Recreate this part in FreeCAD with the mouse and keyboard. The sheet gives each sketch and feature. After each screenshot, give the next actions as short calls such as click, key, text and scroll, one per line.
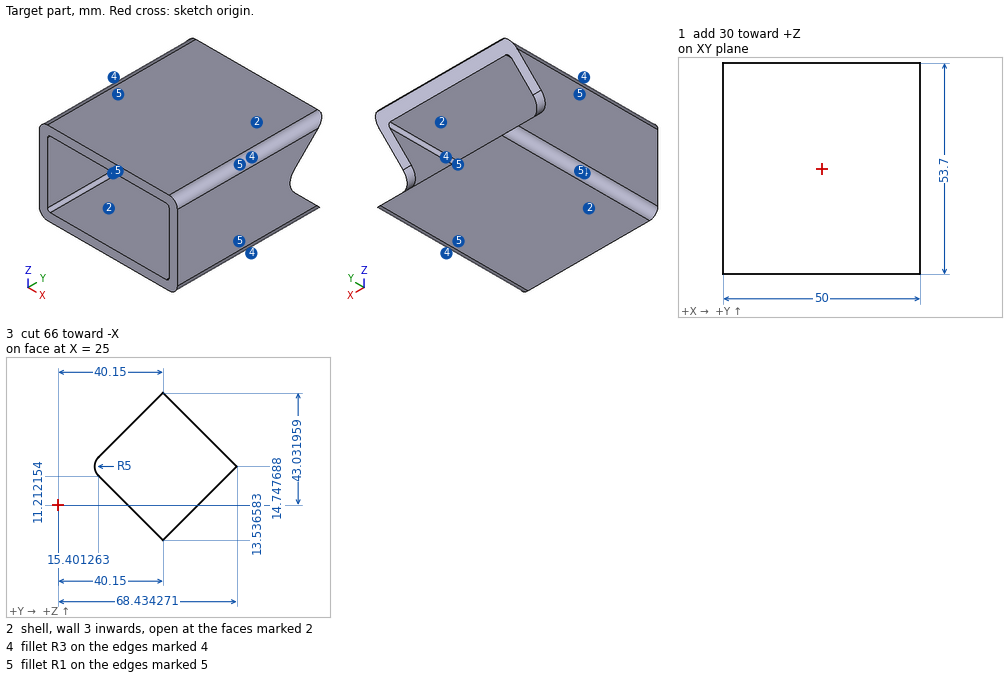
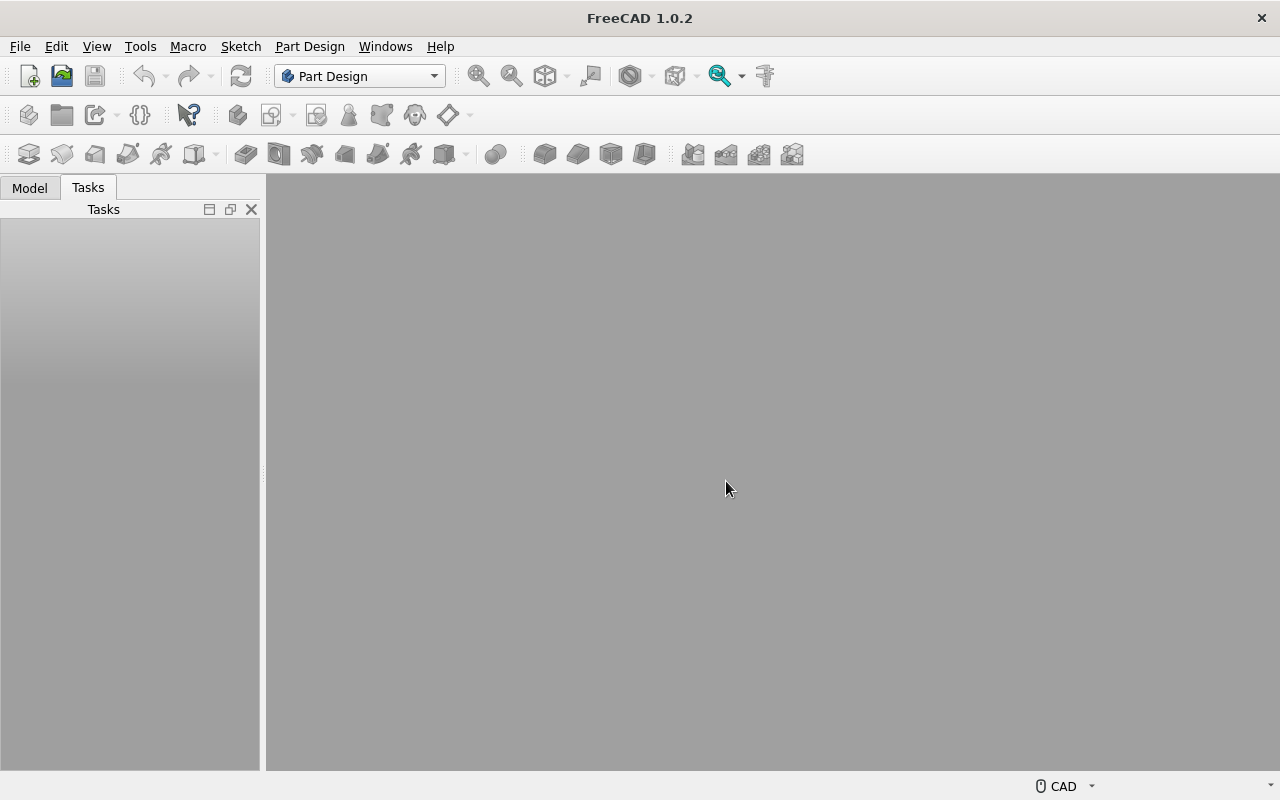
key(ctrl+n)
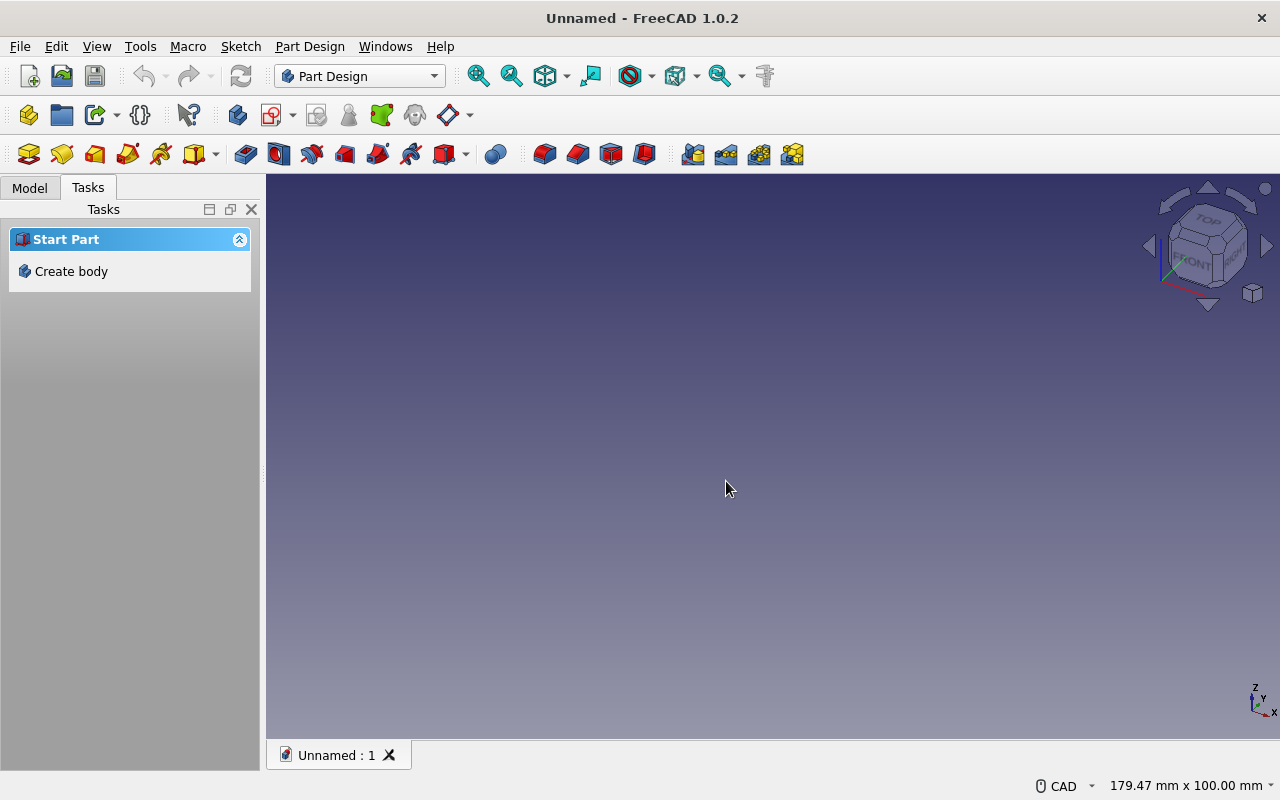
click(270, 116)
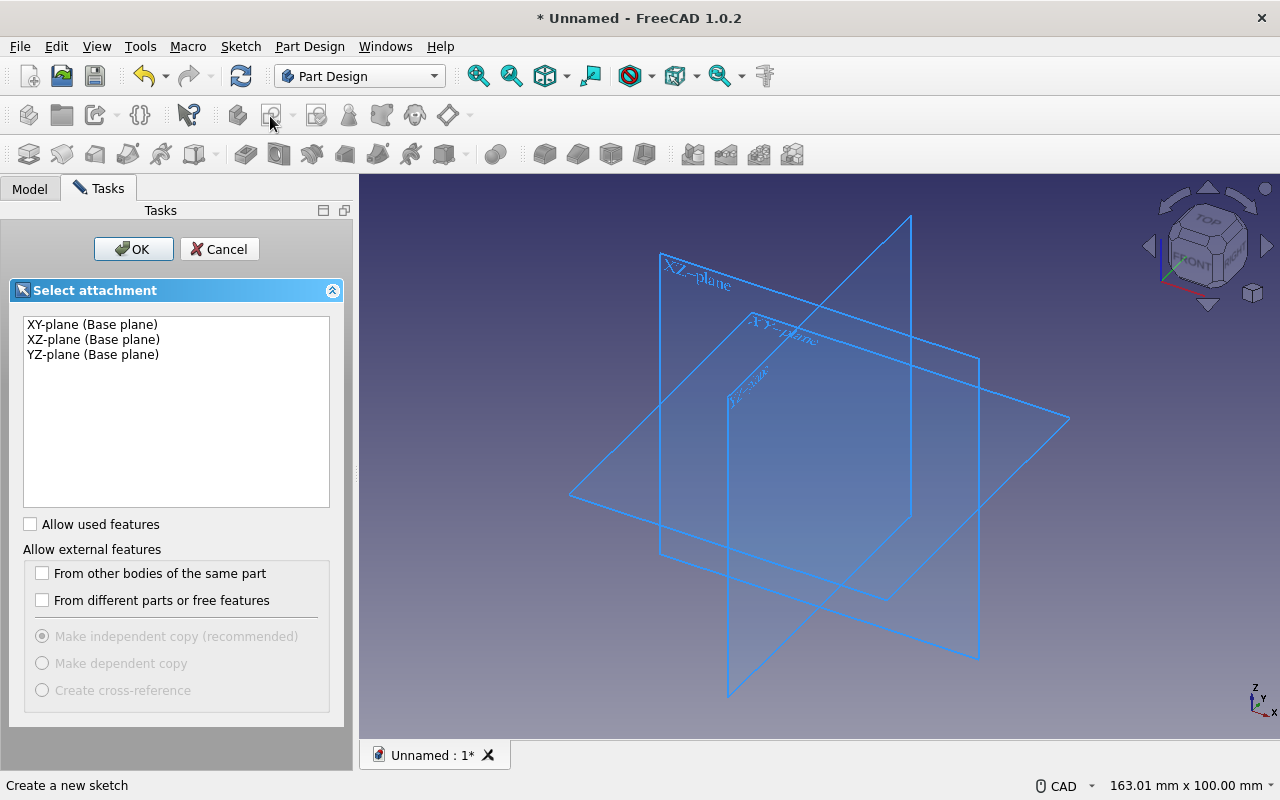
click(84, 324)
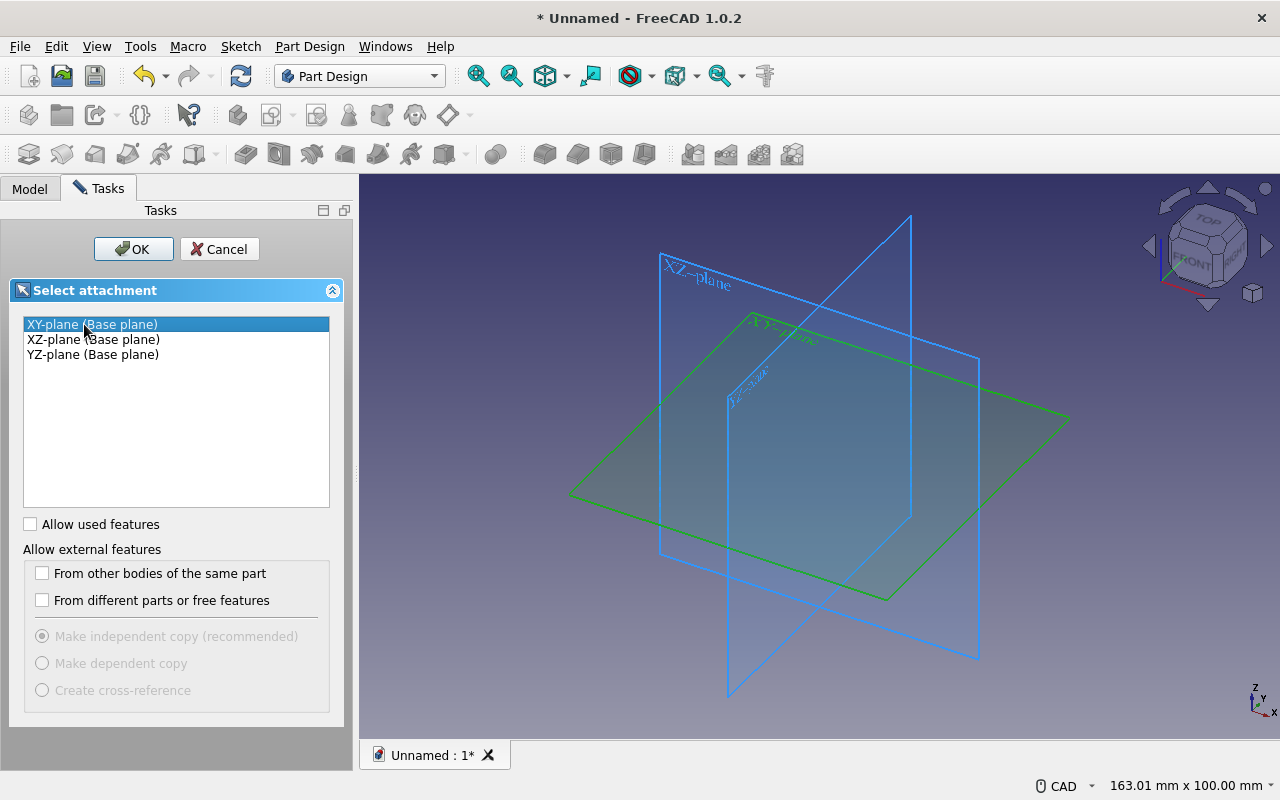
click(134, 249)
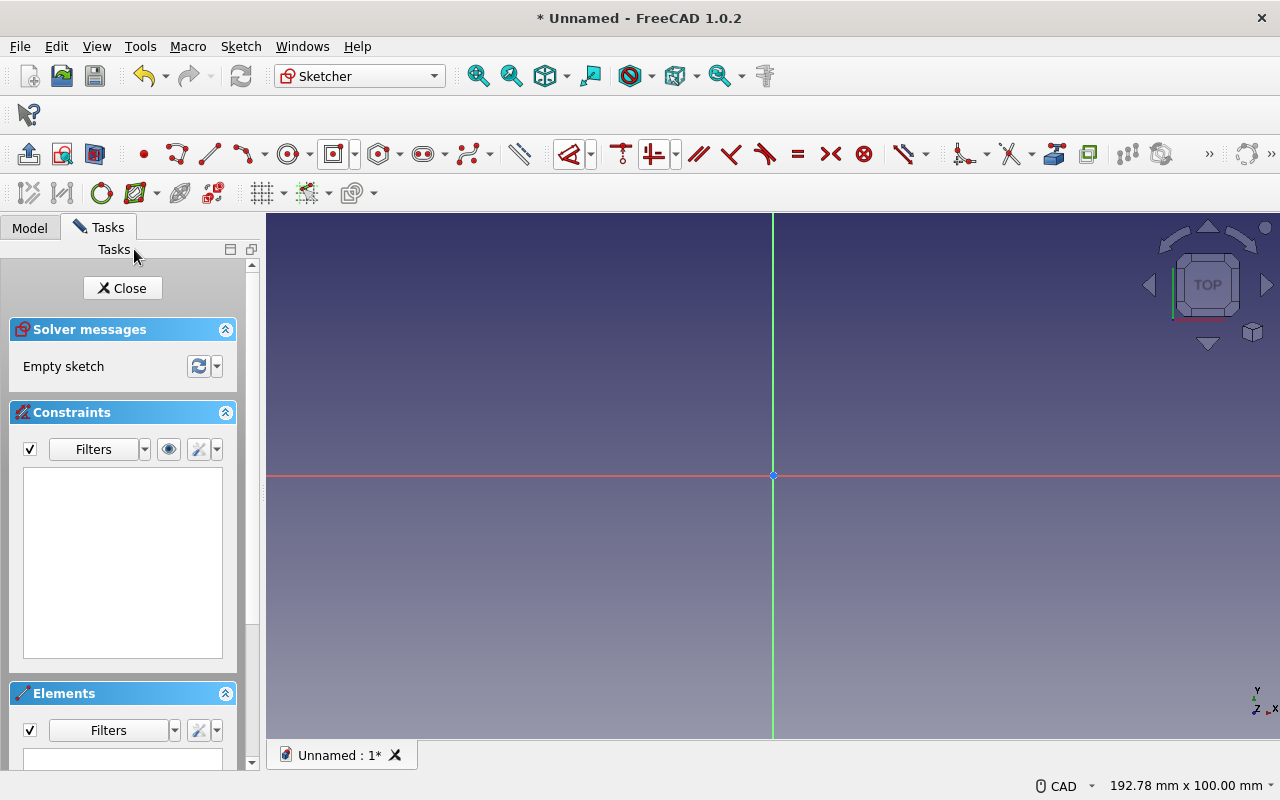
click(332, 154)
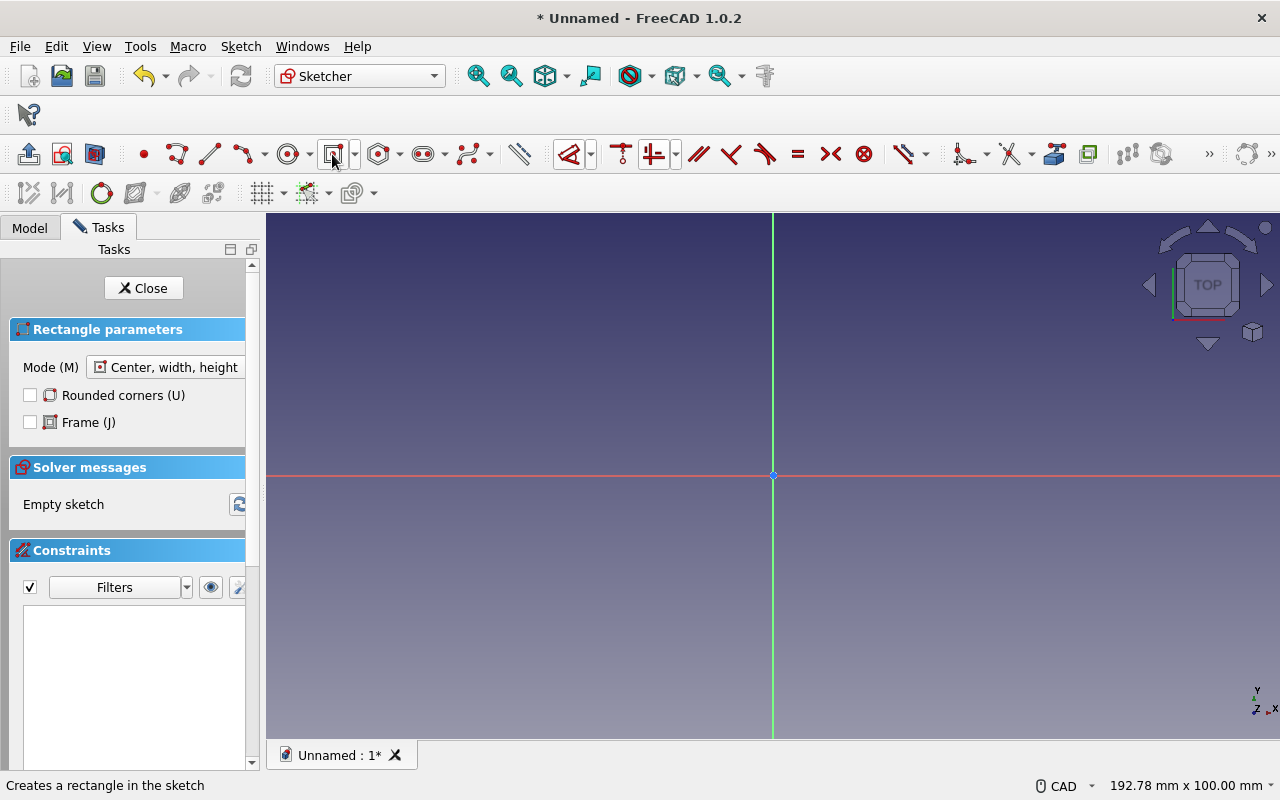
click(773, 476)
move(904, 335)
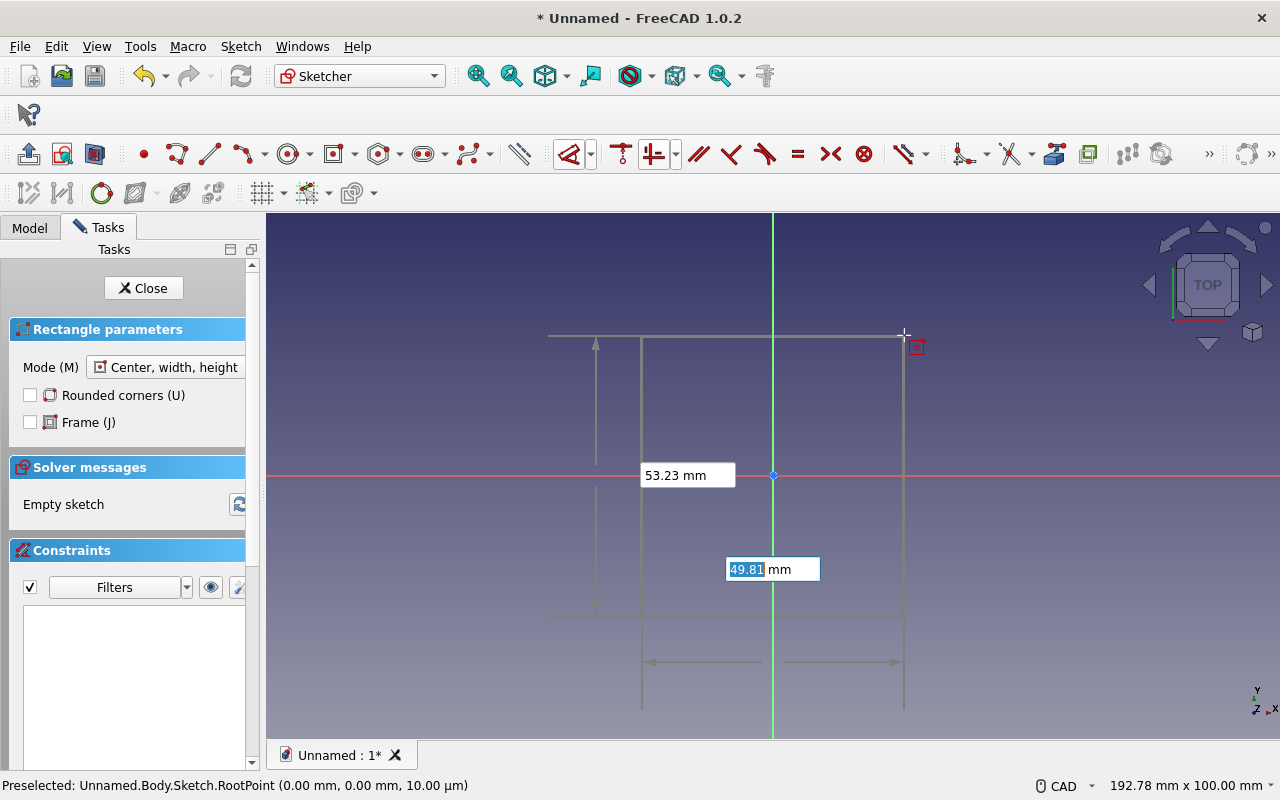
text(50)
key(Tab)
text(53.7)
key(Return)
key(Escape)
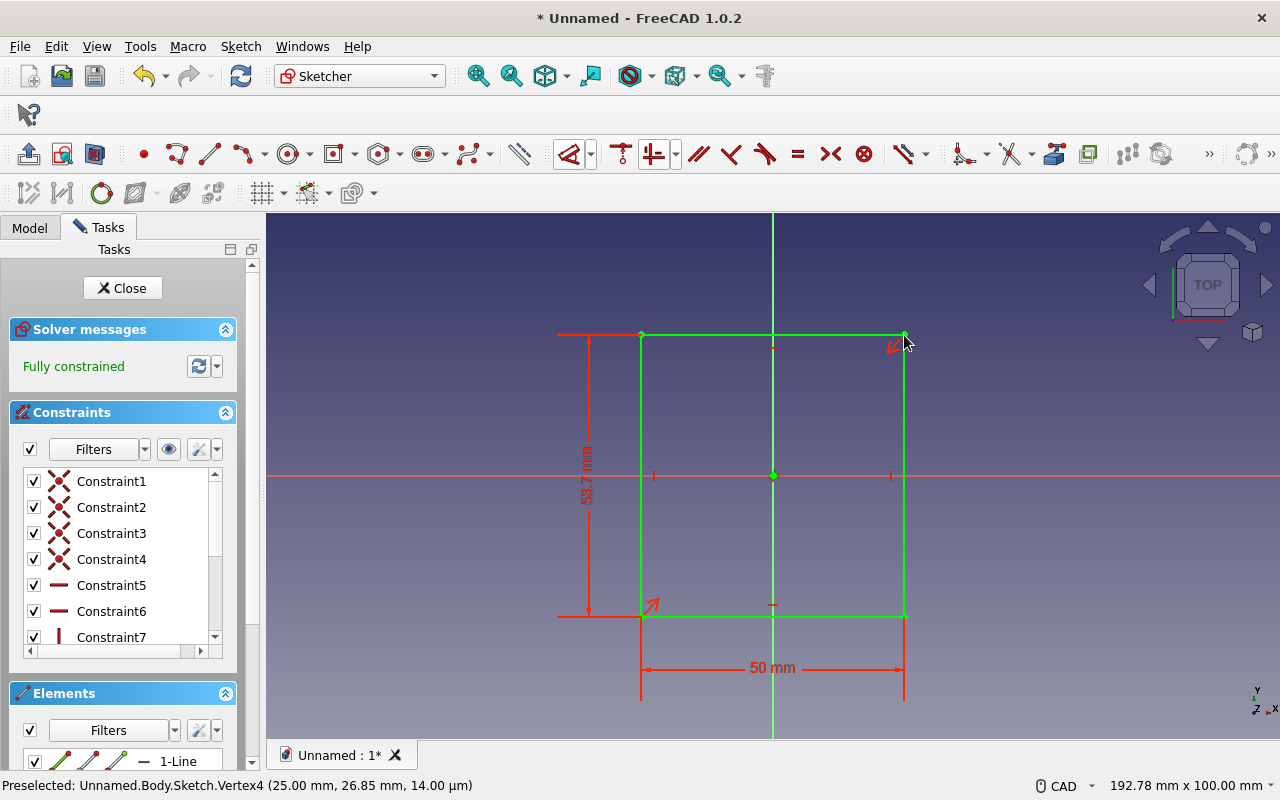
click(123, 288)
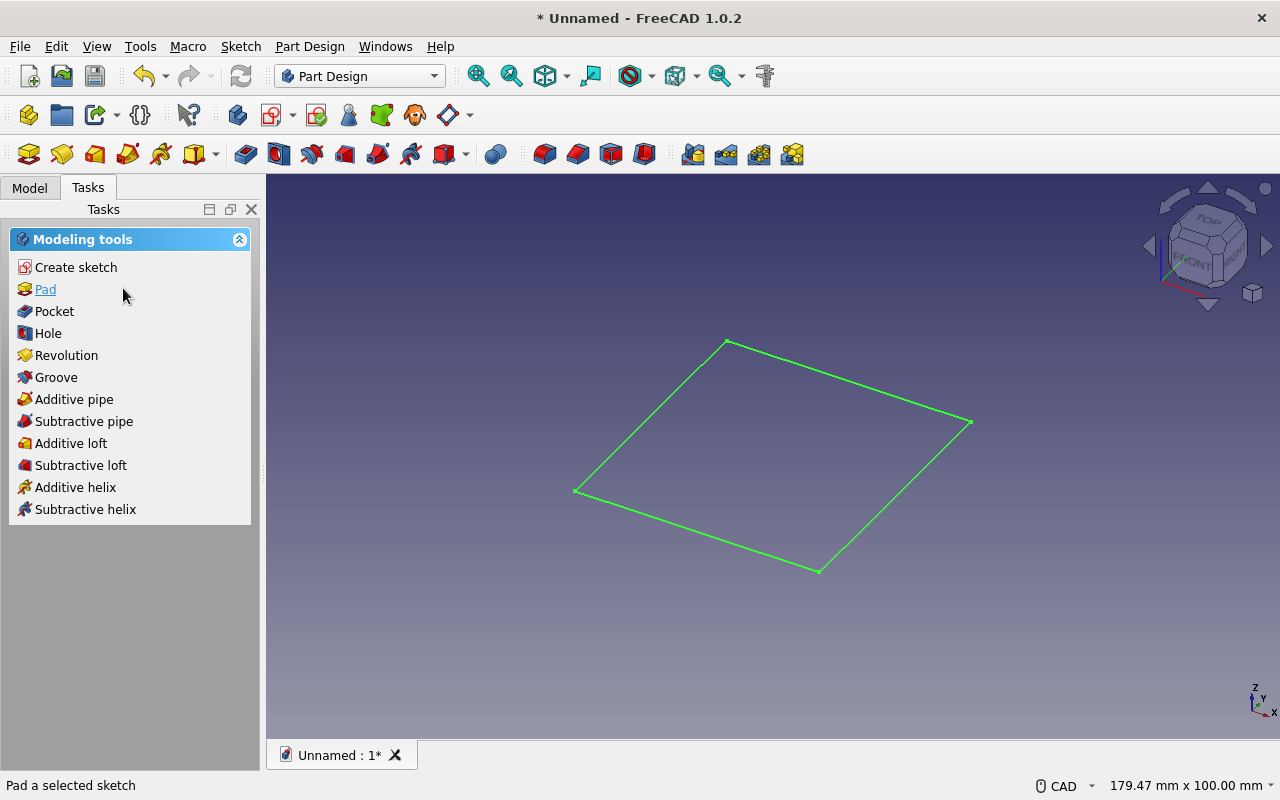
click(29, 154)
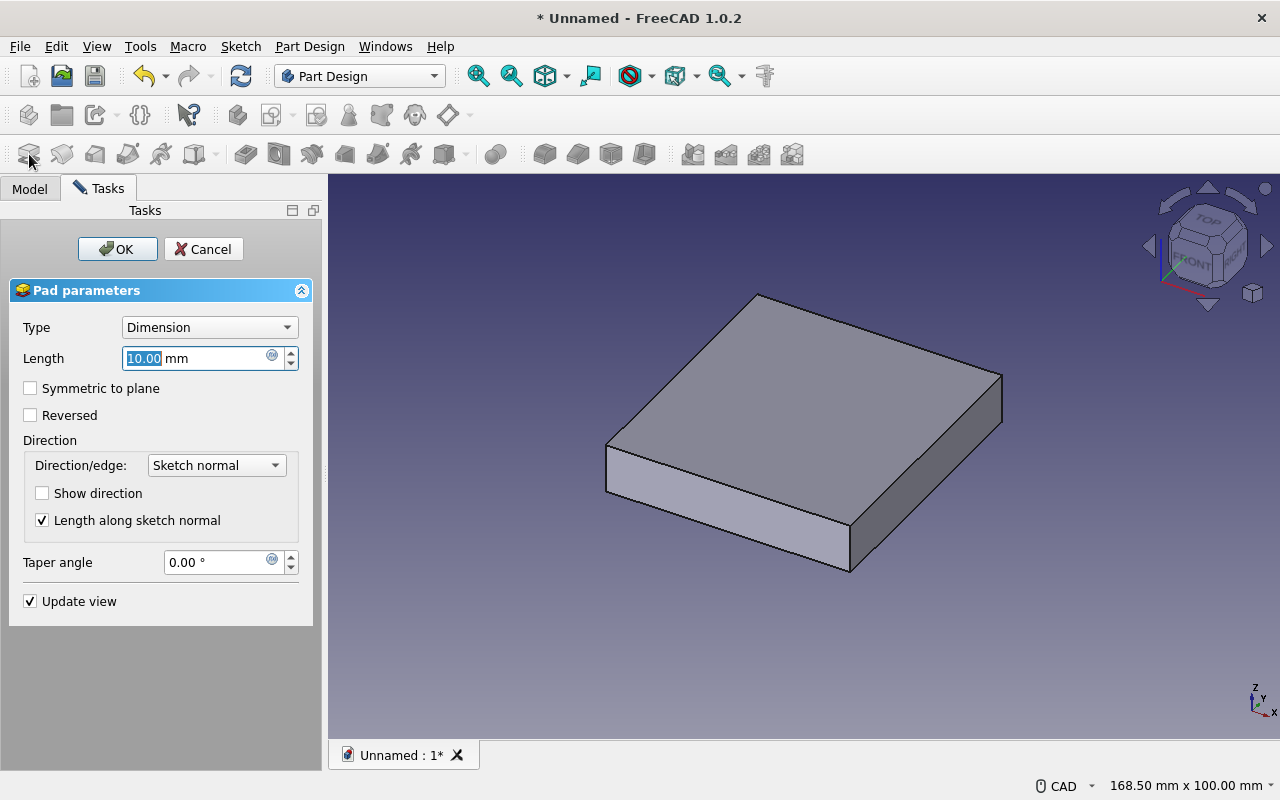
text(30)
key(Tab)